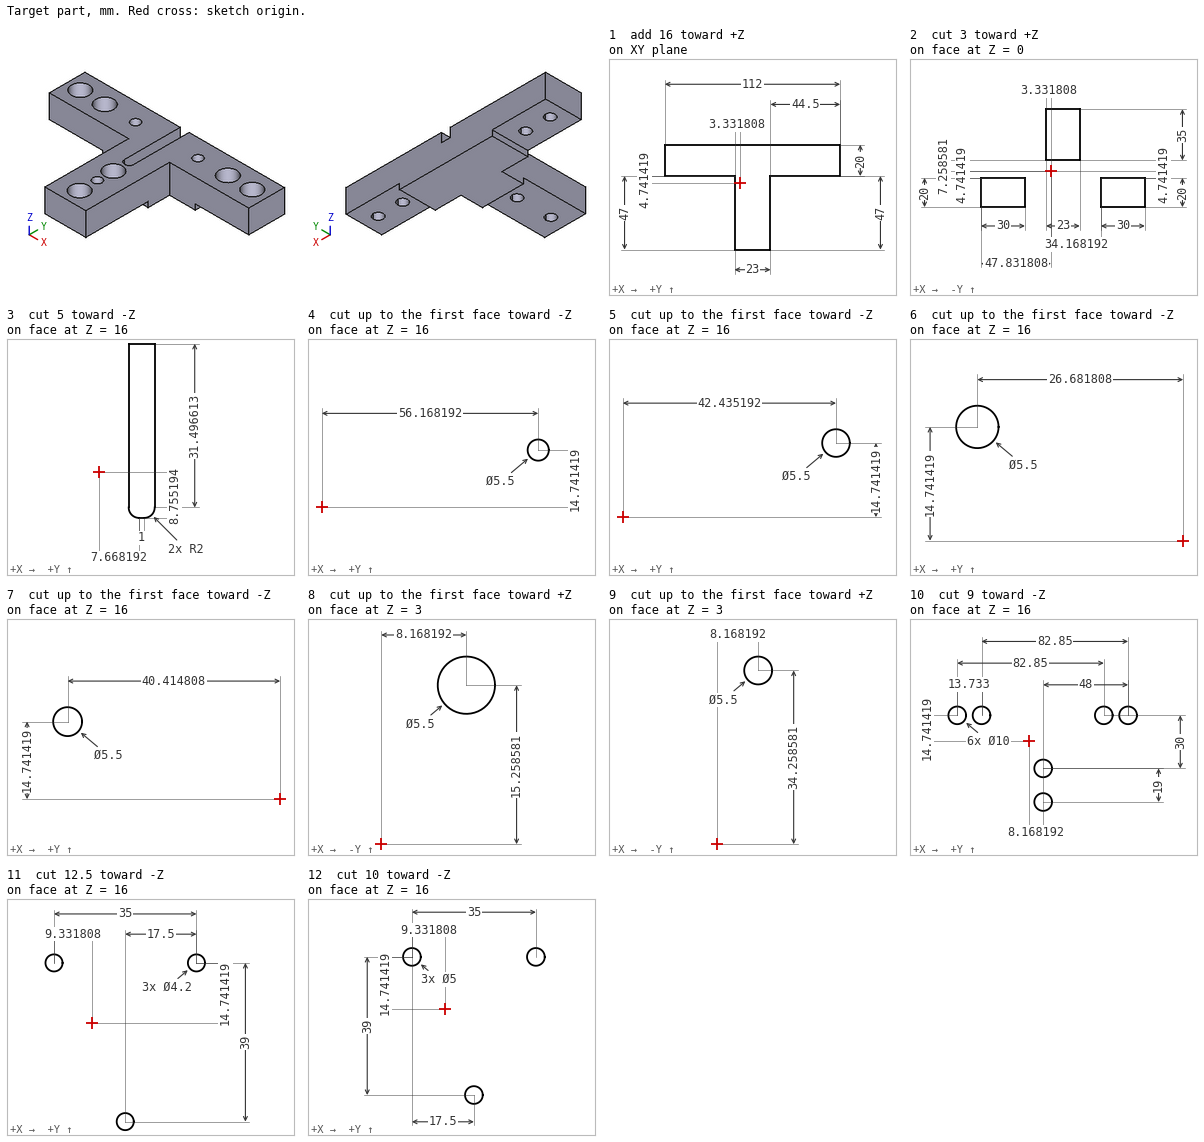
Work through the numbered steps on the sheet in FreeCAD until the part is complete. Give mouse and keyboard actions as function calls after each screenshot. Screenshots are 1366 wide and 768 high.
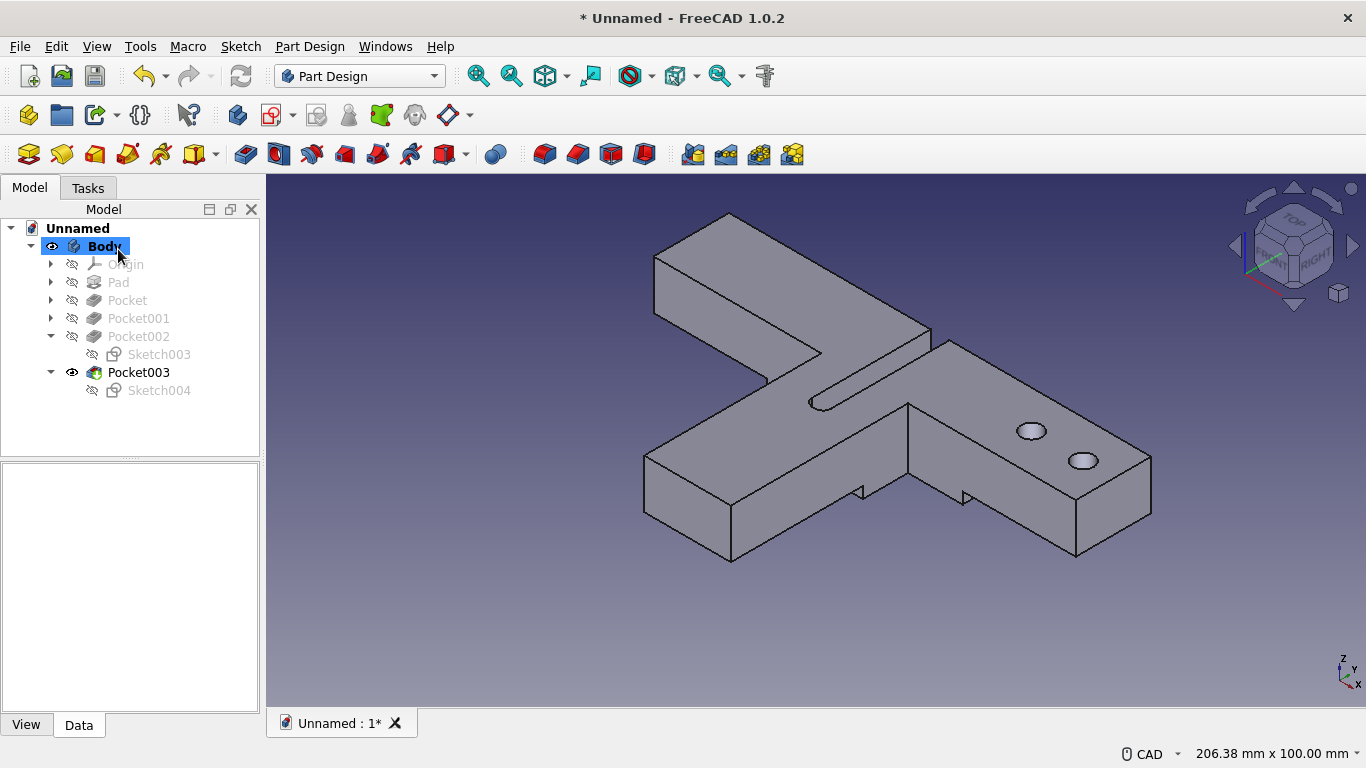
click(742, 448)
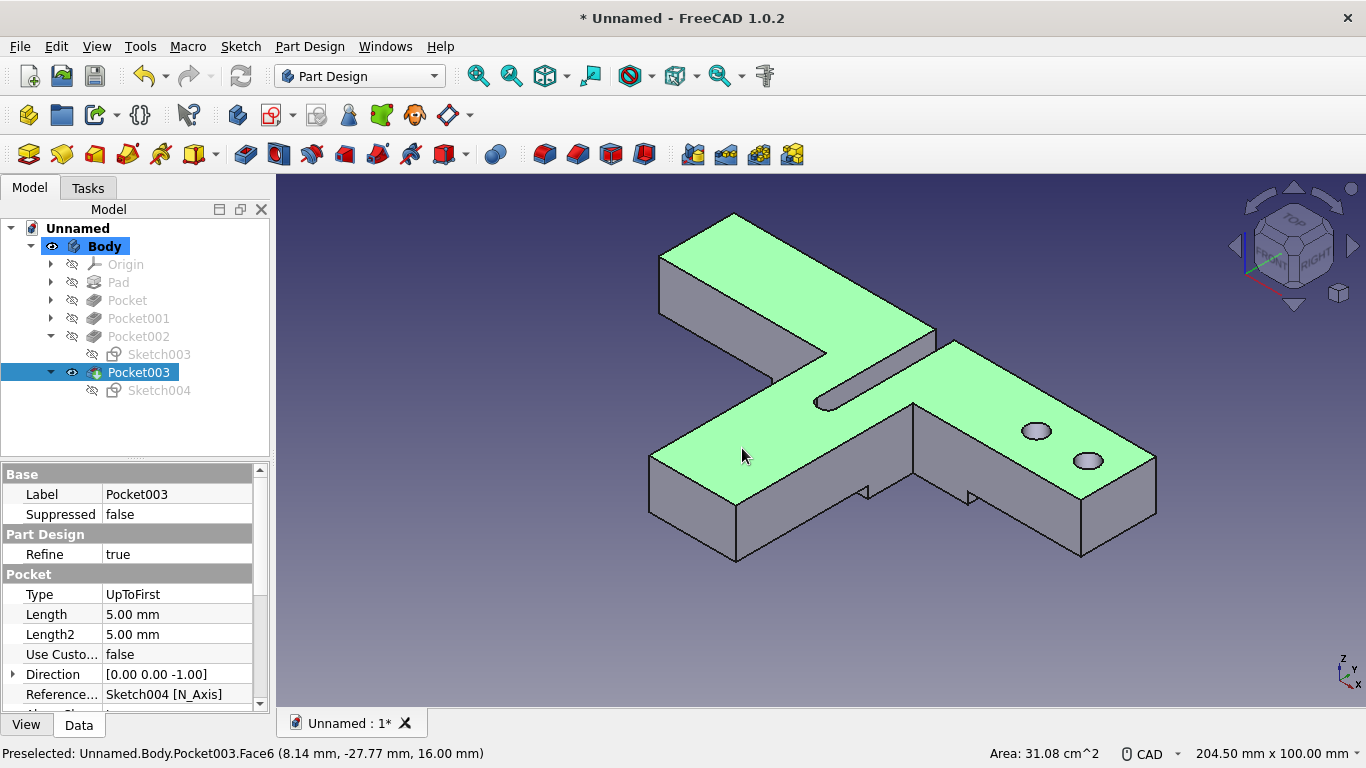
click(270, 116)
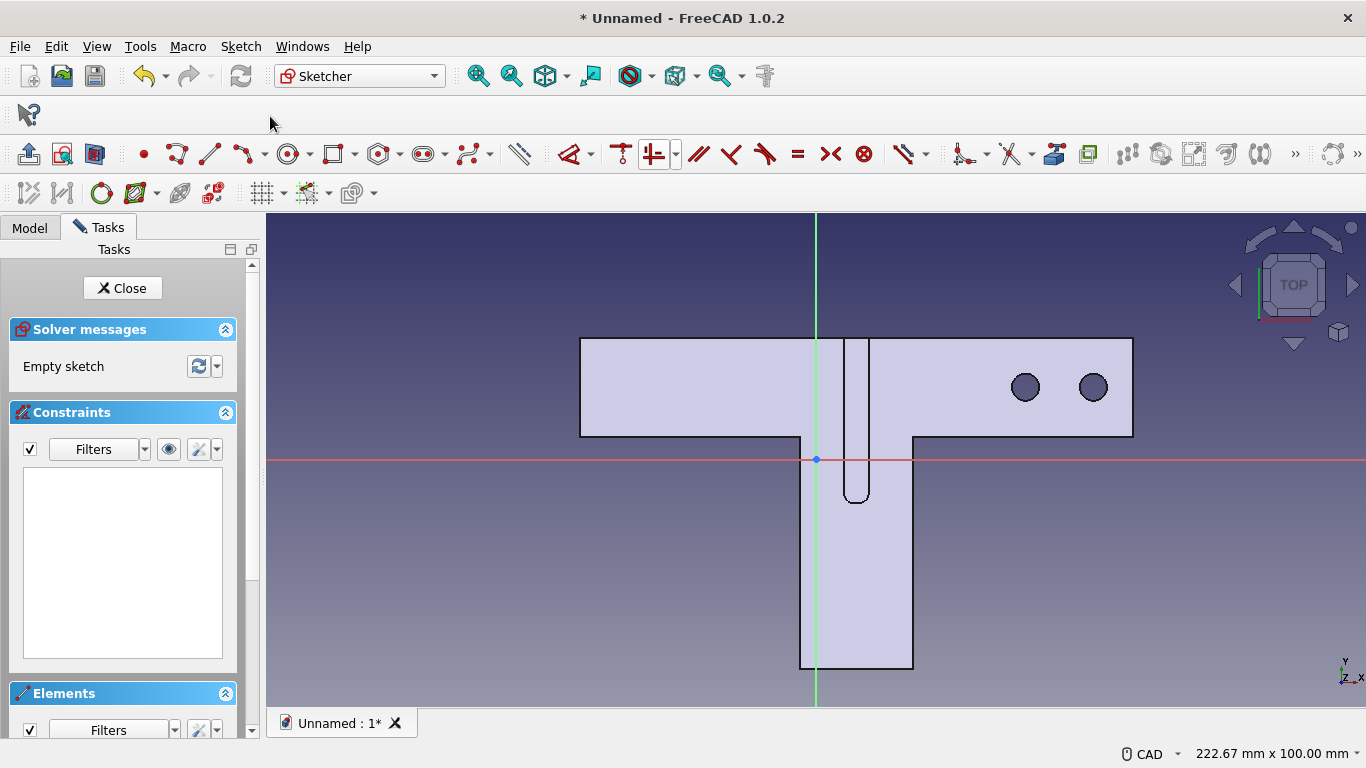
scroll(678, 380, up, 12)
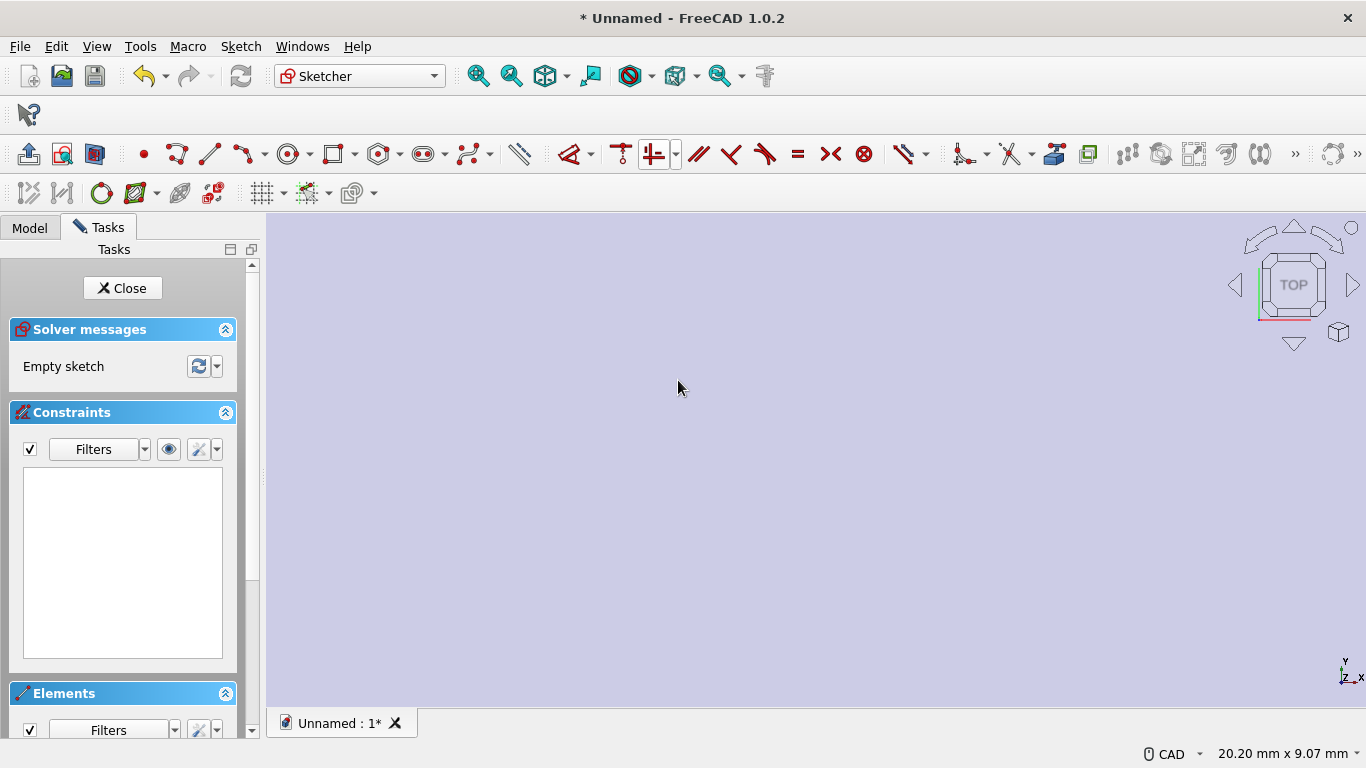
click(288, 154)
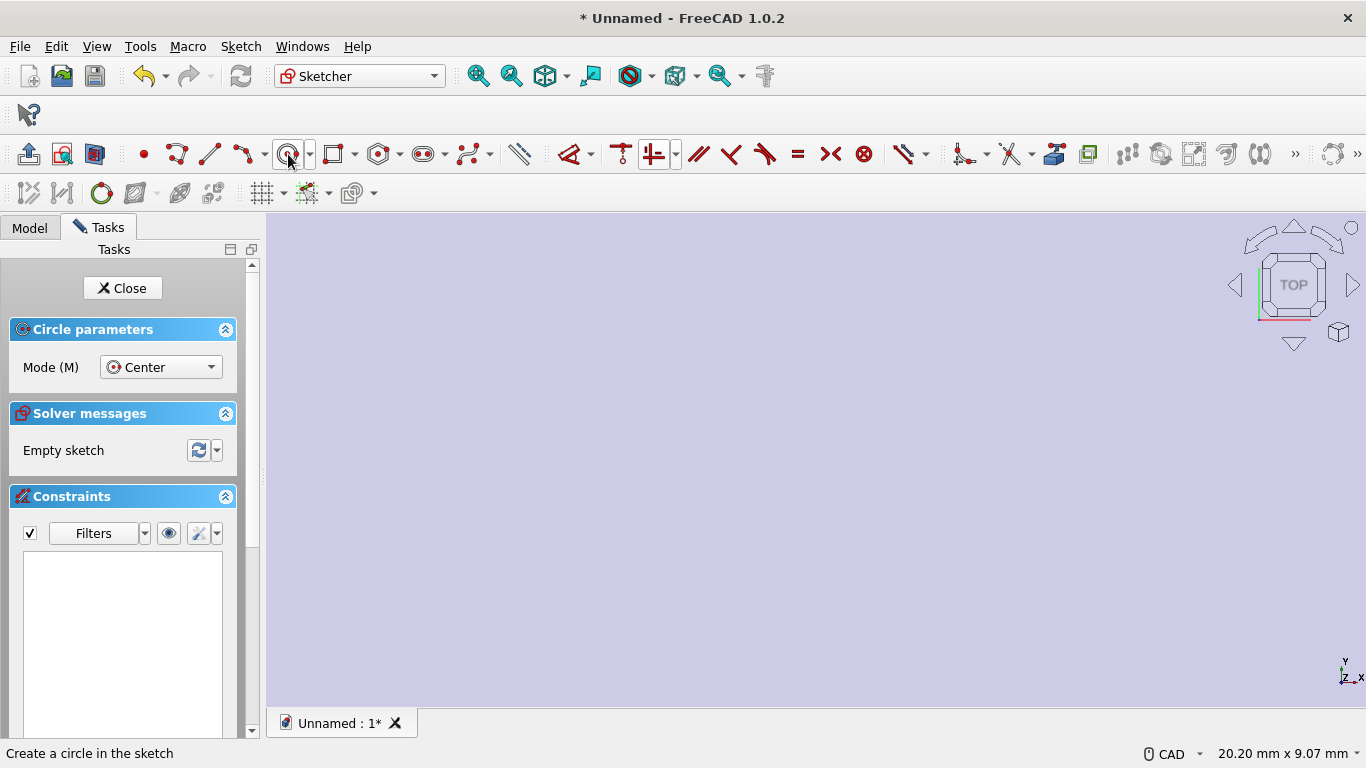
click(742, 456)
move(848, 350)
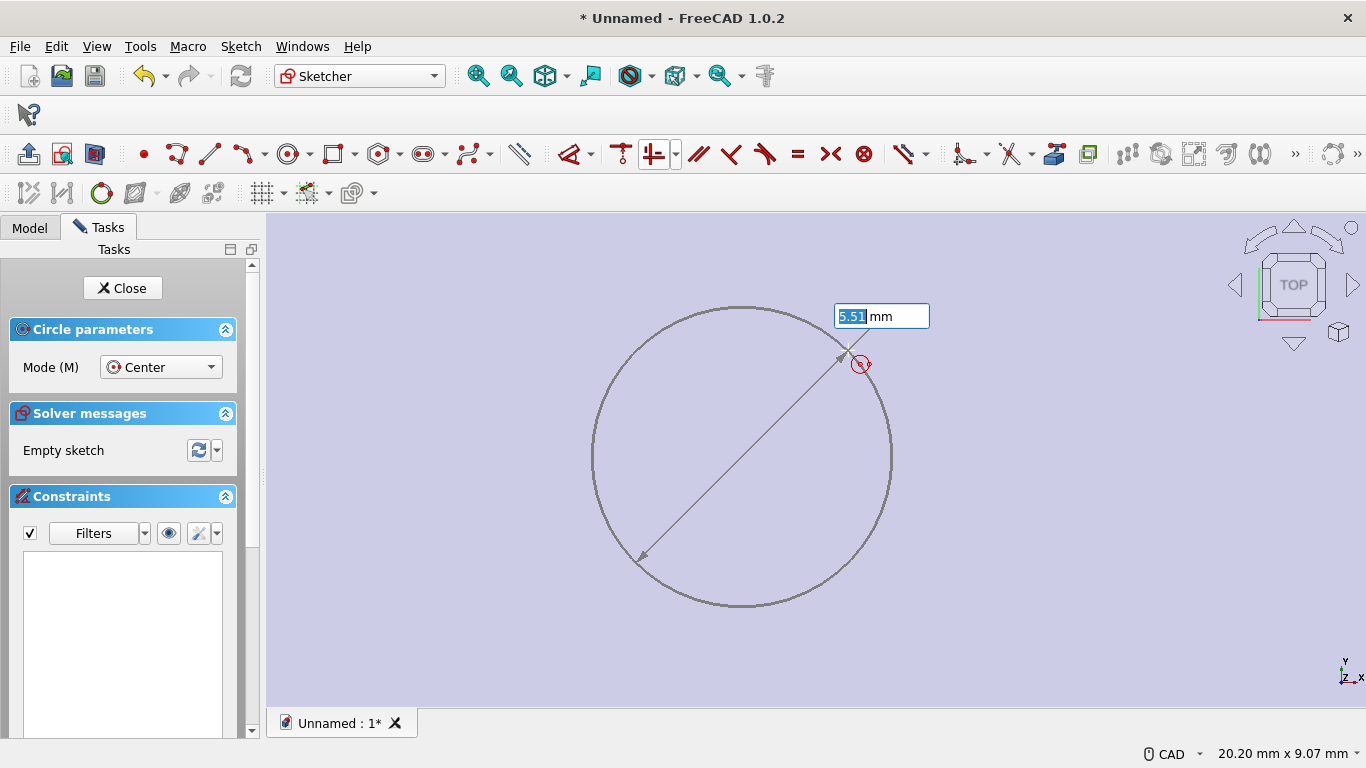
text(5.5)
key(Return)
key(Escape)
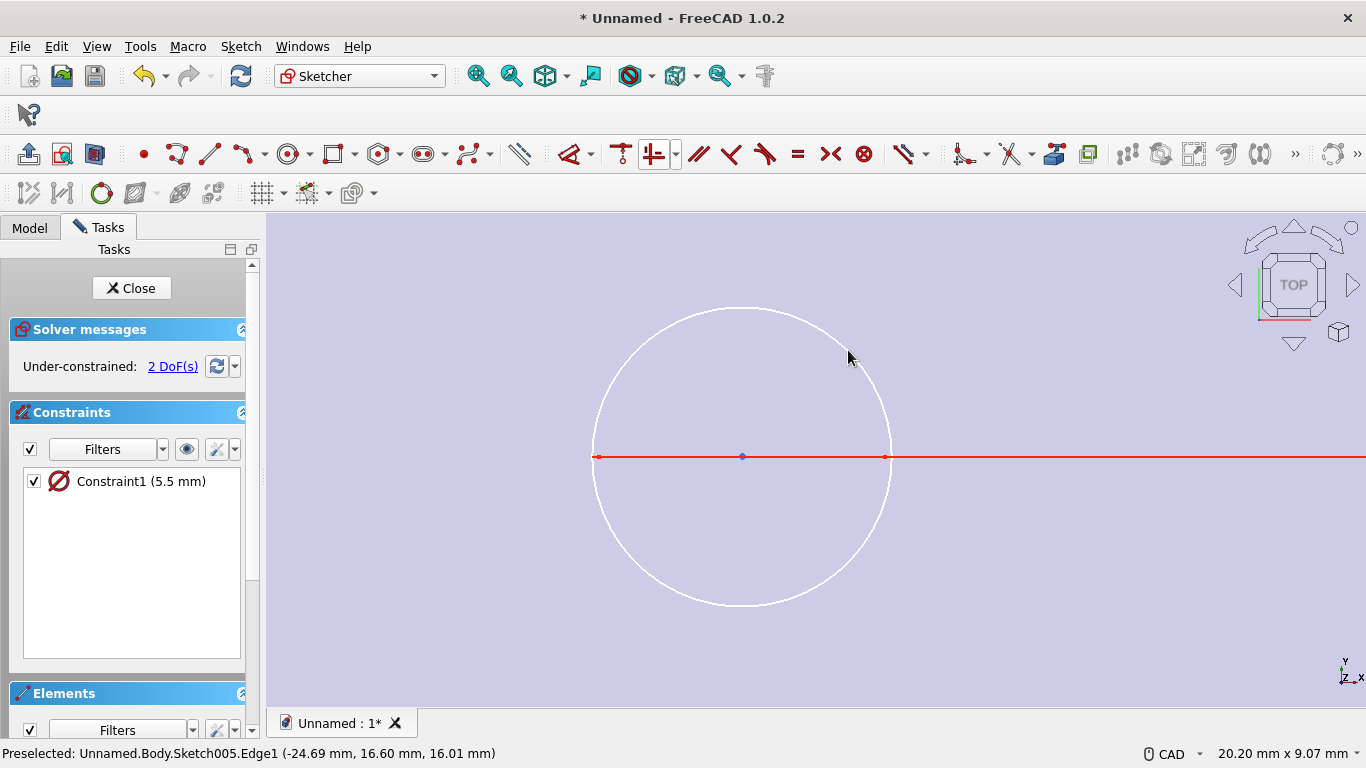
click(568, 154)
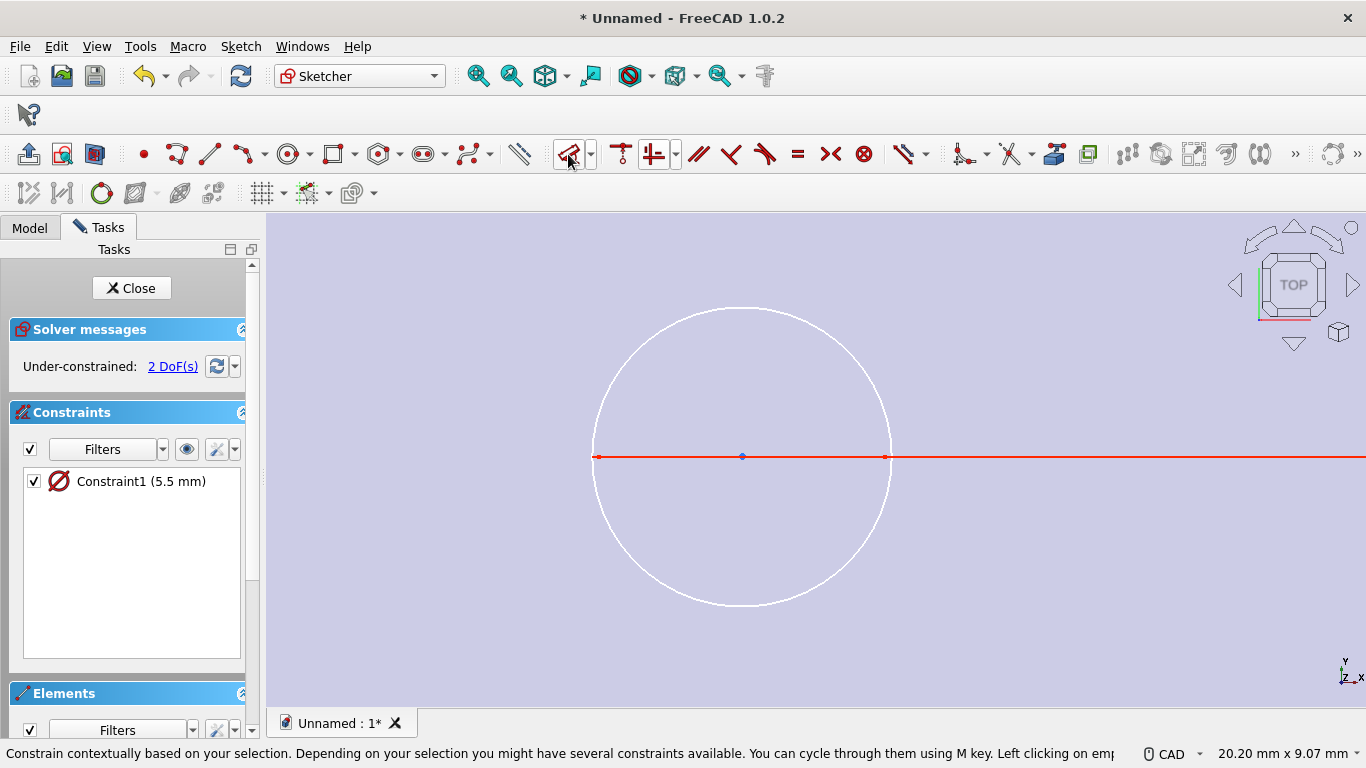
click(742, 457)
click(972, 423)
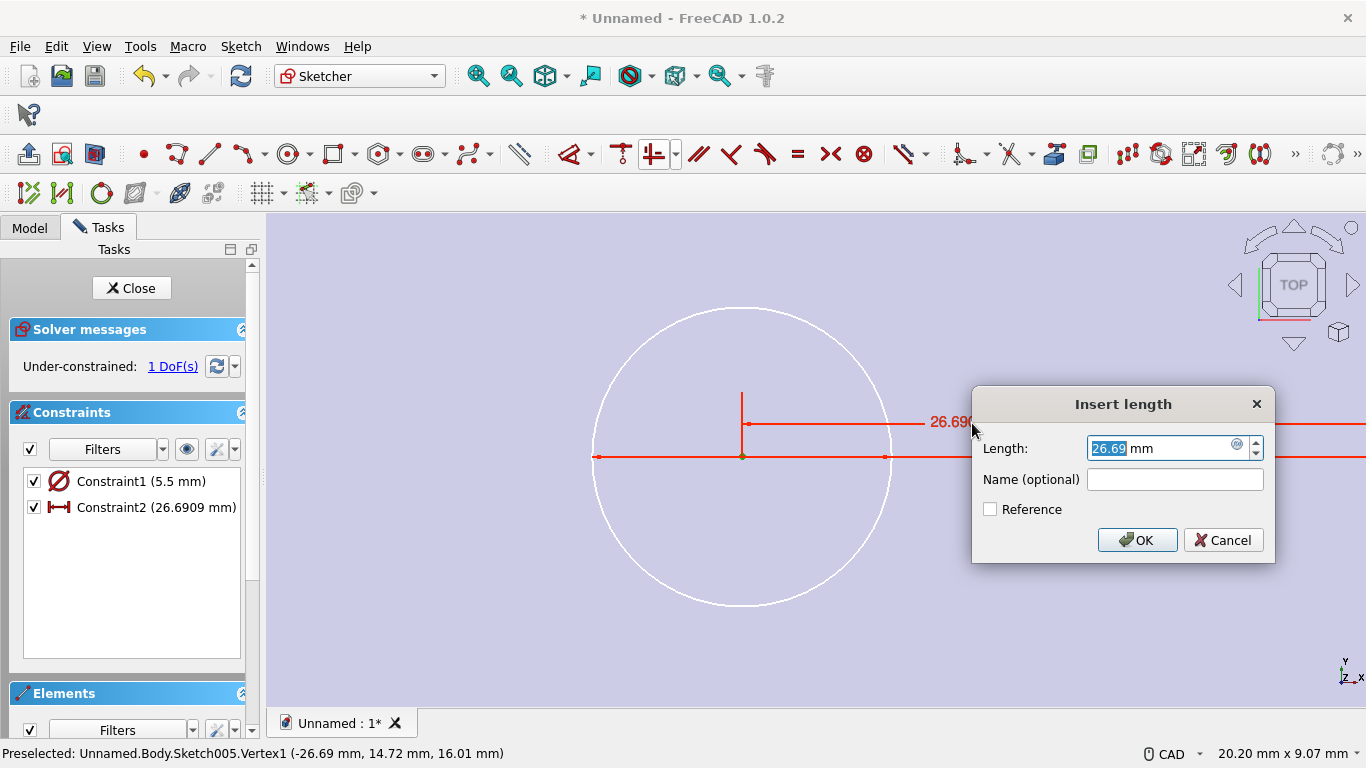
text(26.681808)
key(Return)